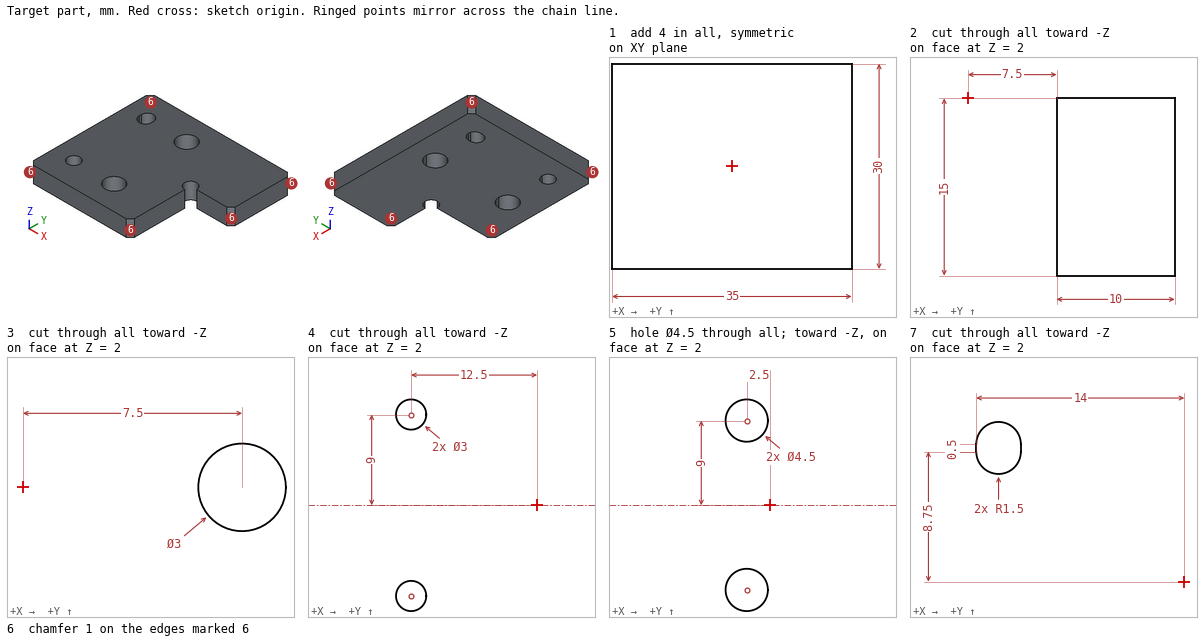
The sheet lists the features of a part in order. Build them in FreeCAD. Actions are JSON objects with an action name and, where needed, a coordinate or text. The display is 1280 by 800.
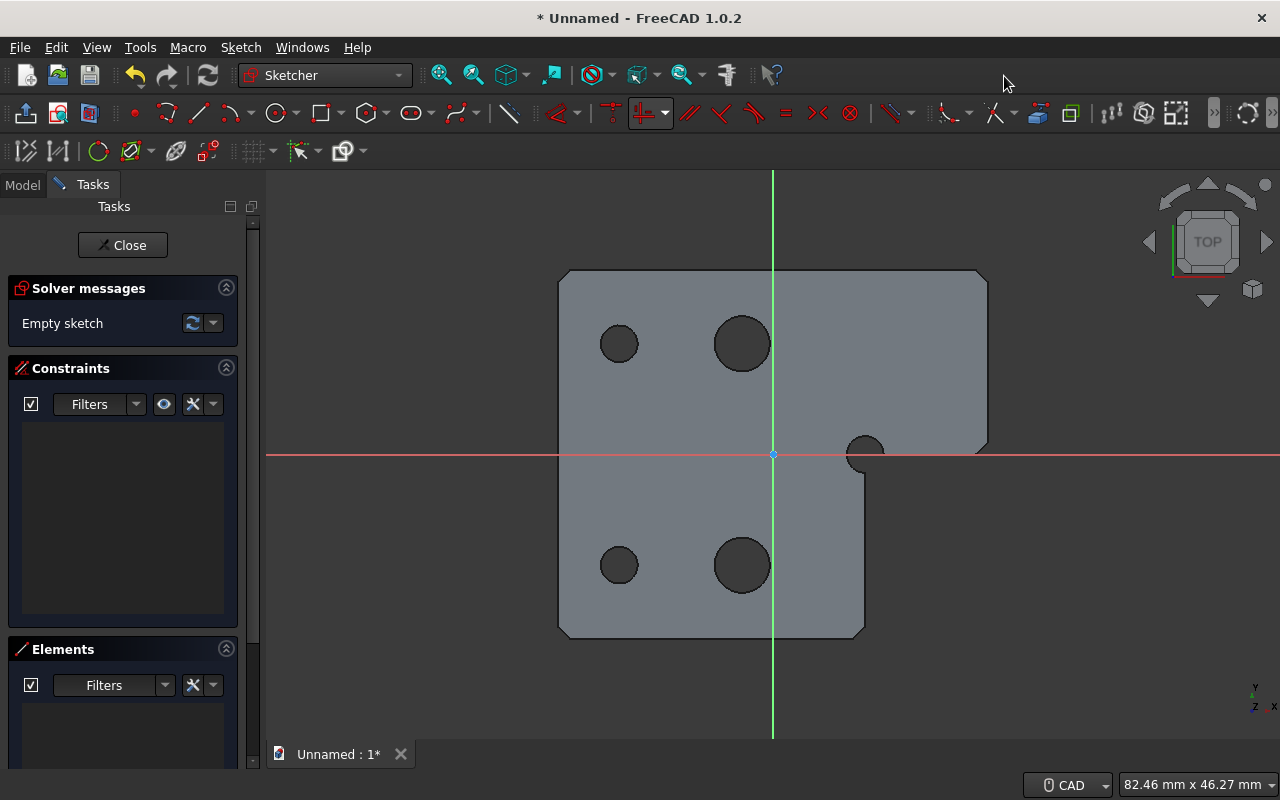
{"action": "scroll", "coordinate": [609, 330], "scroll_direction": "up", "scroll_amount": 11}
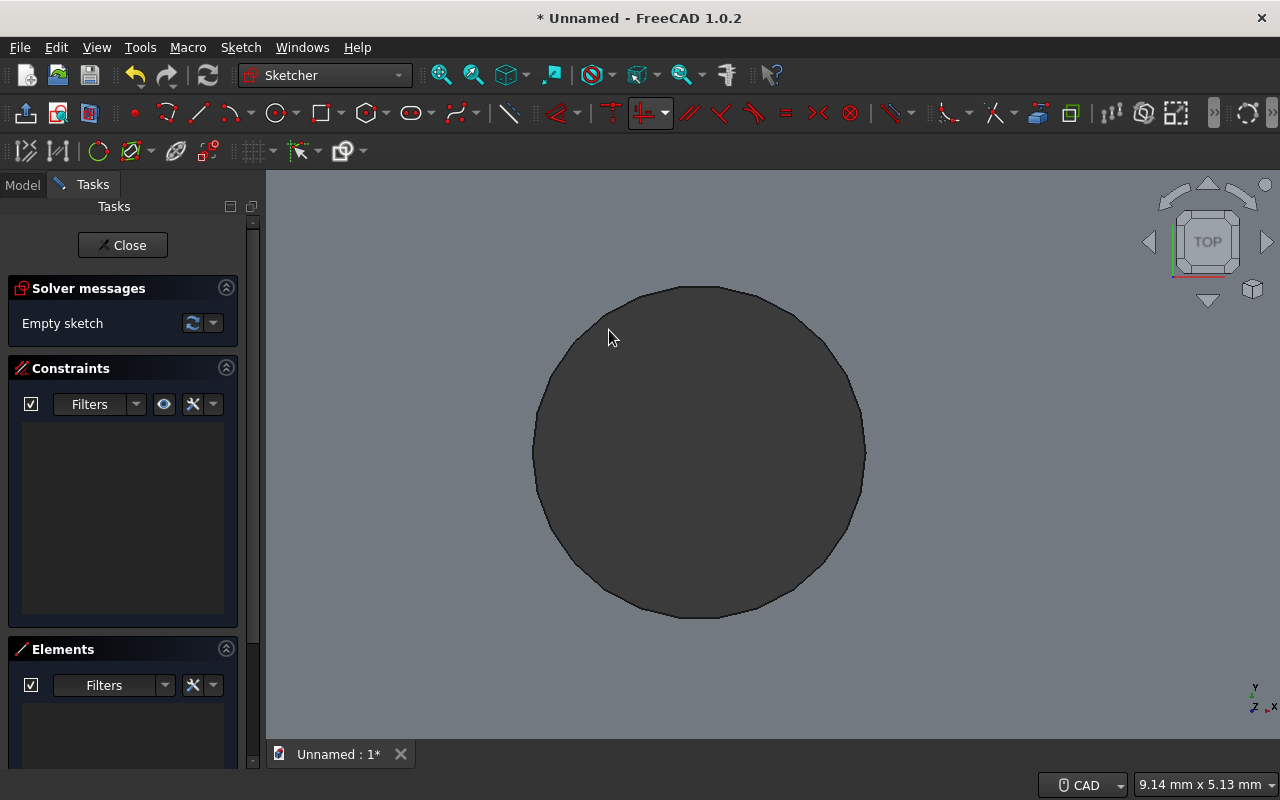
{"action": "key", "text": "g s"}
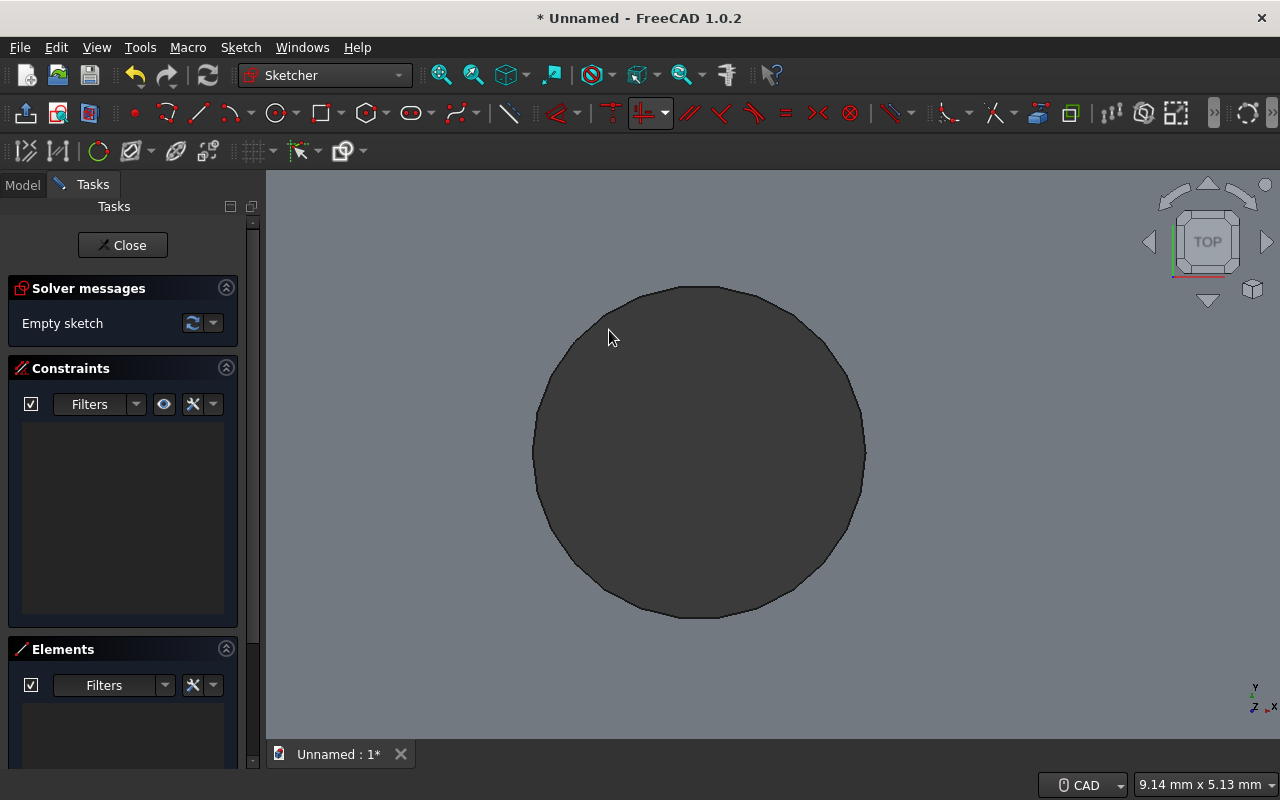
{"action": "left_click", "coordinate": [699, 480]}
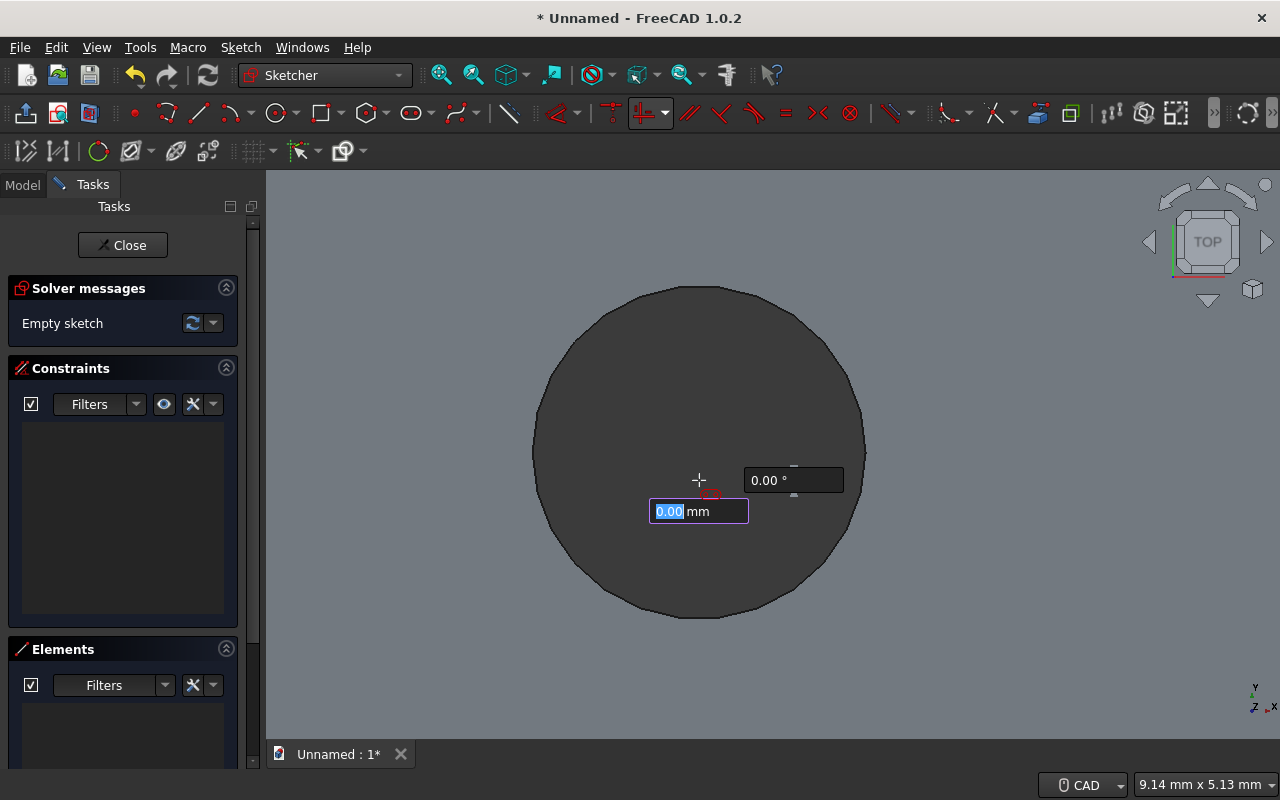
{"action": "left_click", "coordinate": [699, 425]}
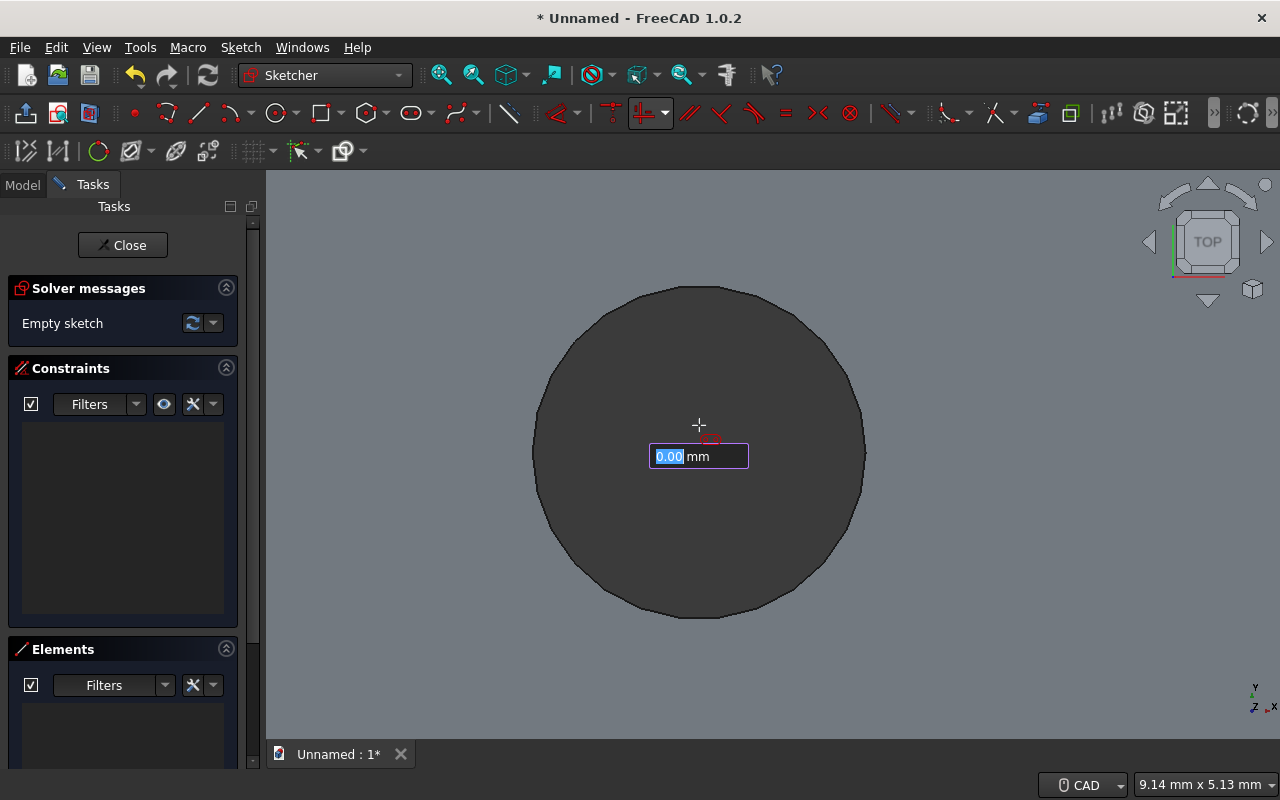
{"action": "left_click", "coordinate": [866, 453]}
{"action": "key", "text": "Escape"}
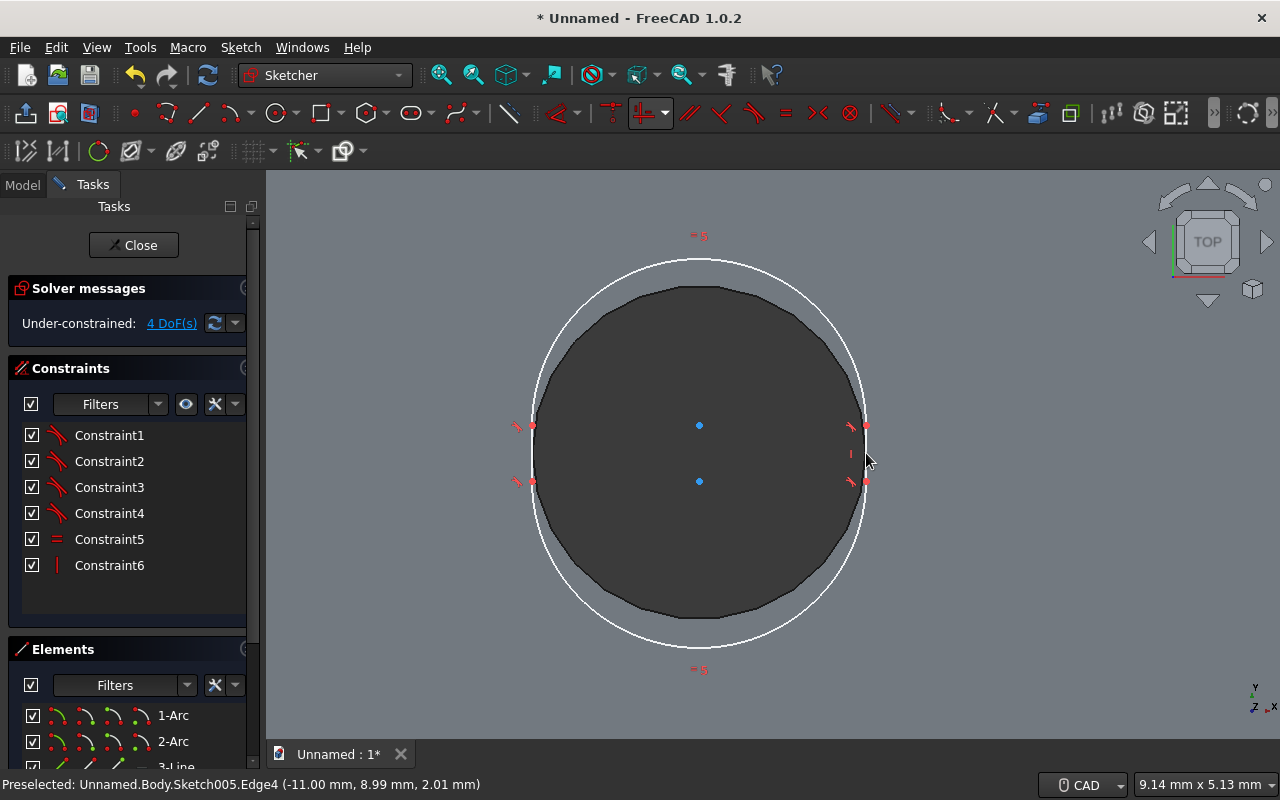
{"action": "key", "text": "d"}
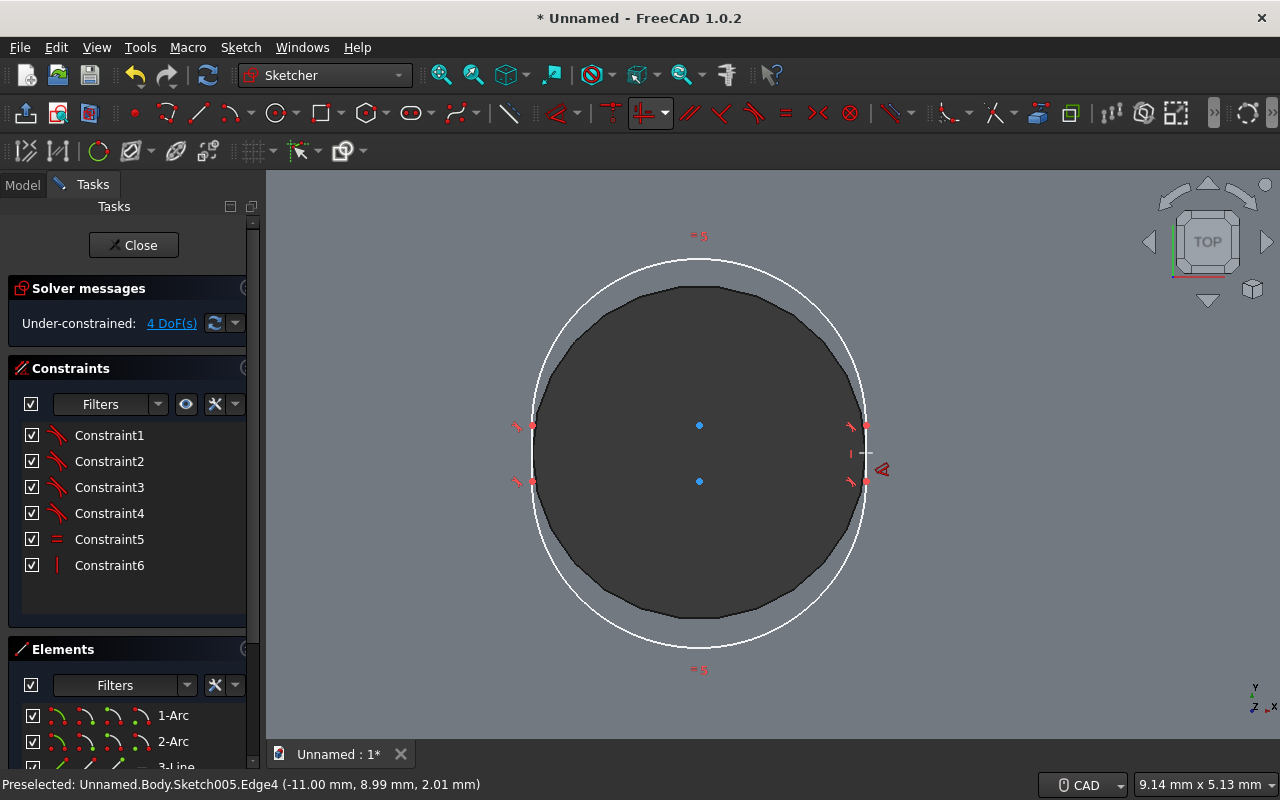
{"action": "left_click", "coordinate": [601, 616]}
{"action": "left_click", "coordinate": [582, 642]}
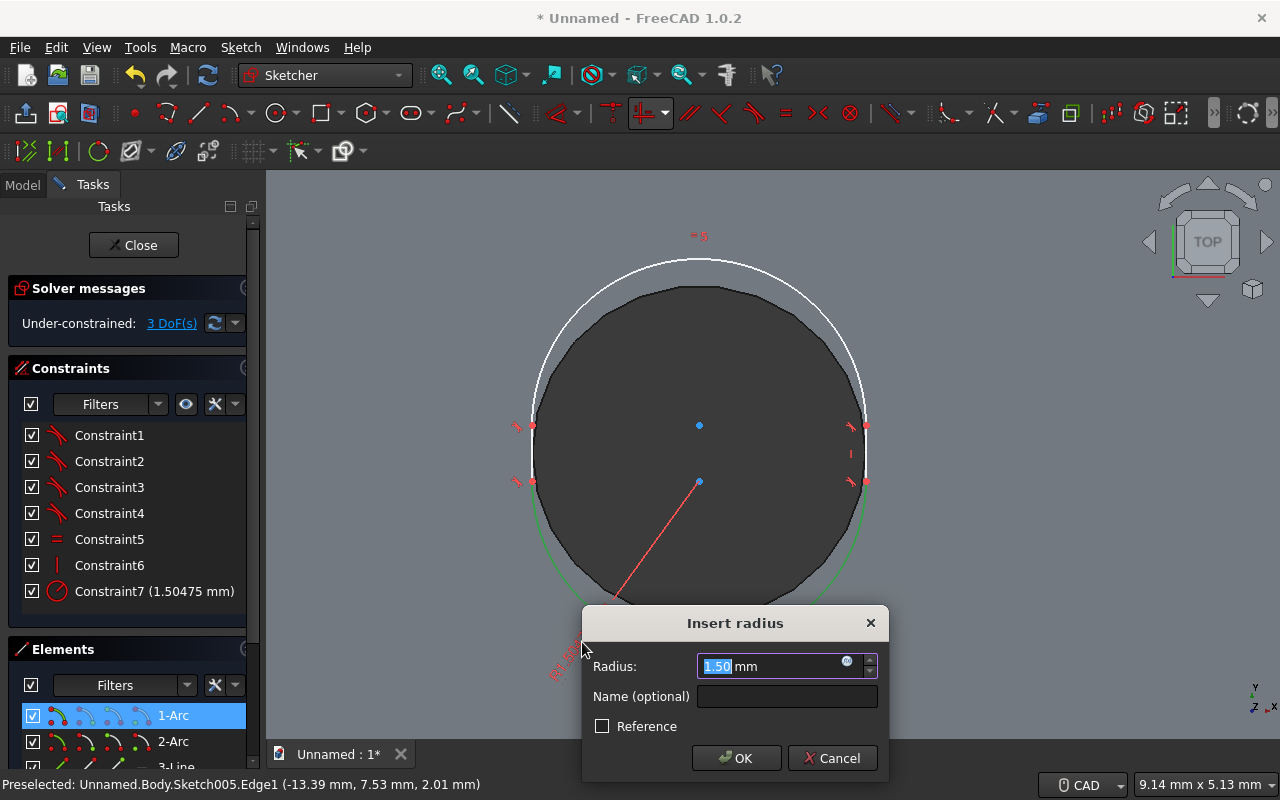
{"action": "type", "text": "1.5"}
{"action": "key", "text": "Return"}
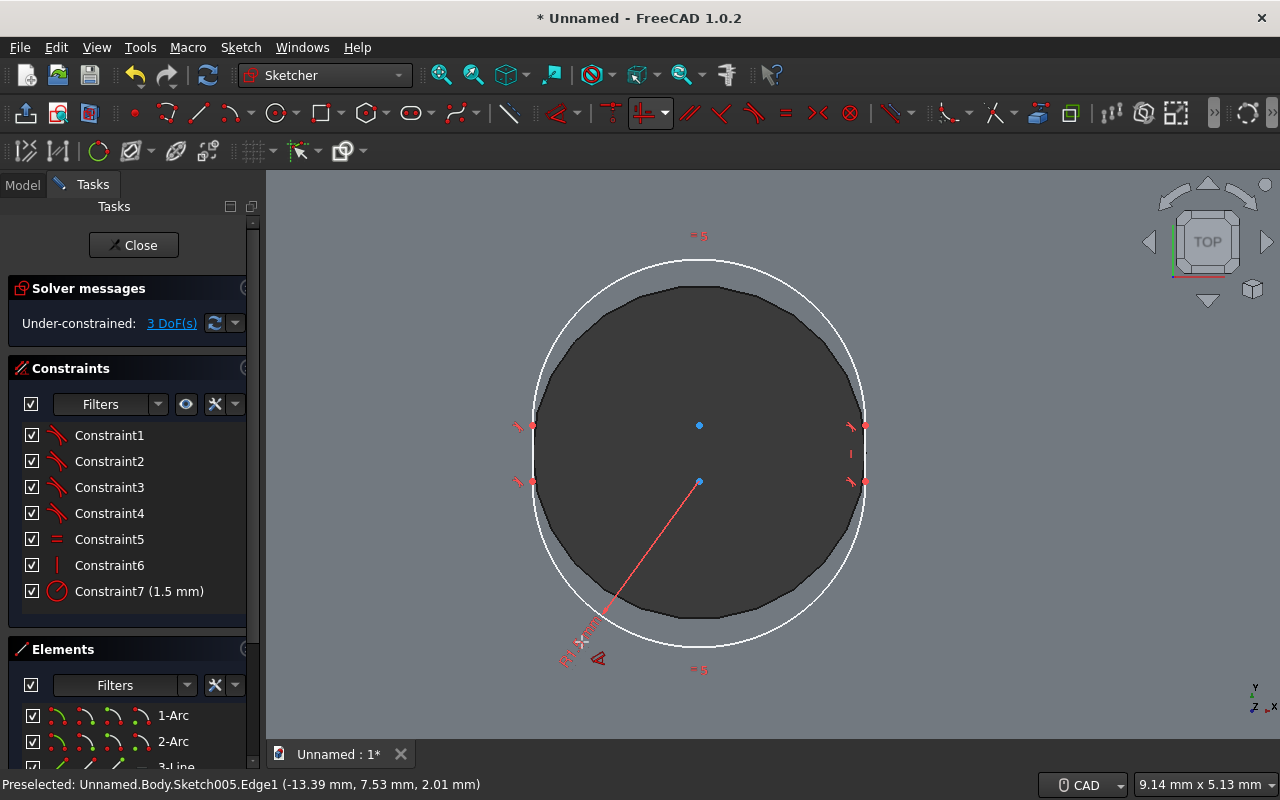
{"action": "left_click", "coordinate": [533, 465]}
{"action": "left_click", "coordinate": [499, 454]}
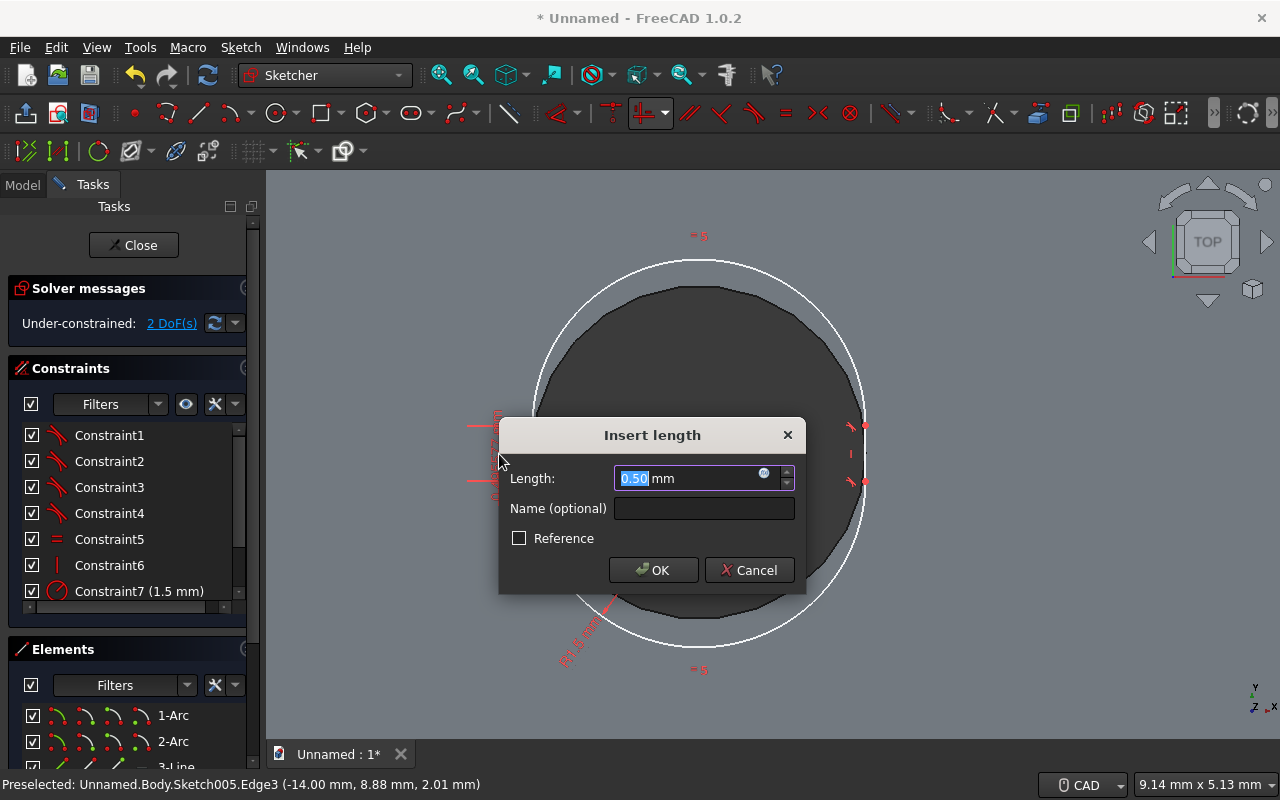
{"action": "type", "text": "0.5"}
{"action": "key", "text": "Return"}